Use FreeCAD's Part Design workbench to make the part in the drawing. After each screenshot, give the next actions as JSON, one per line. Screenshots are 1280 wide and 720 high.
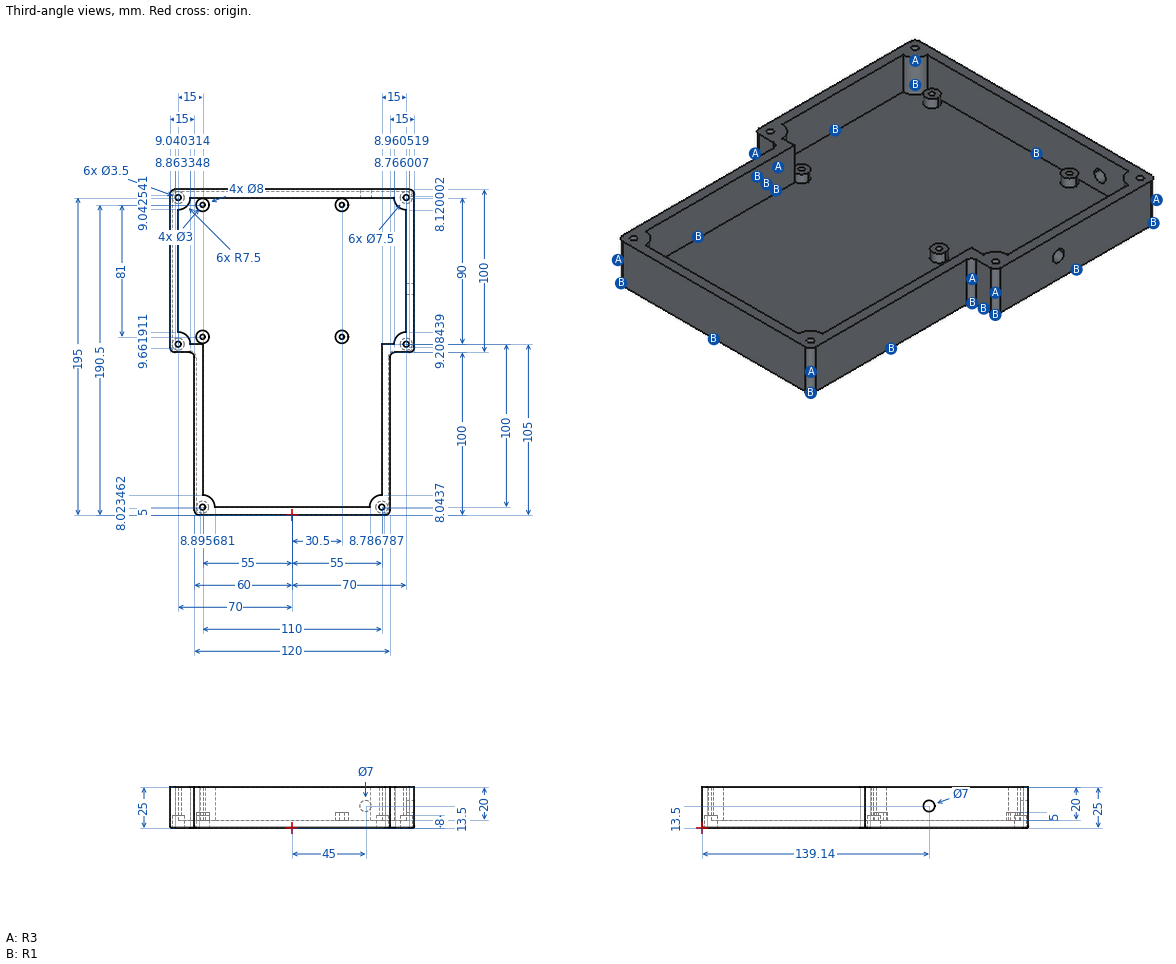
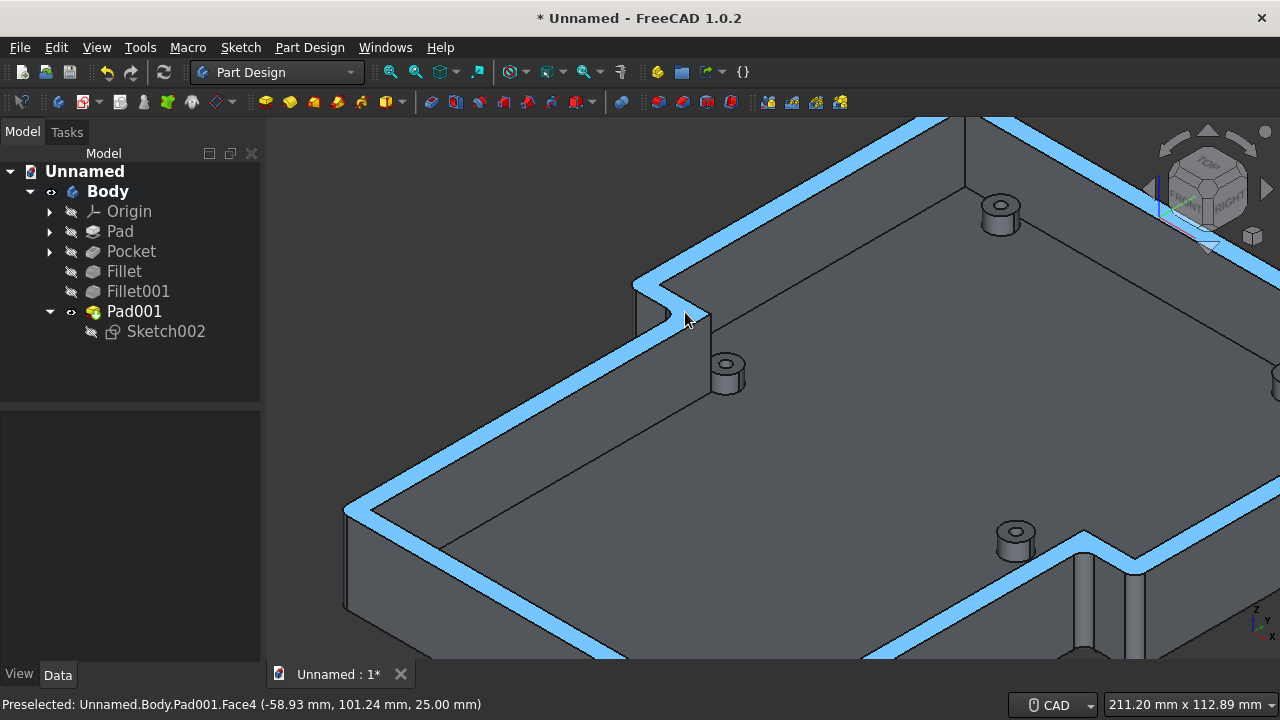
{"action": "left_click", "coordinate": [684, 313]}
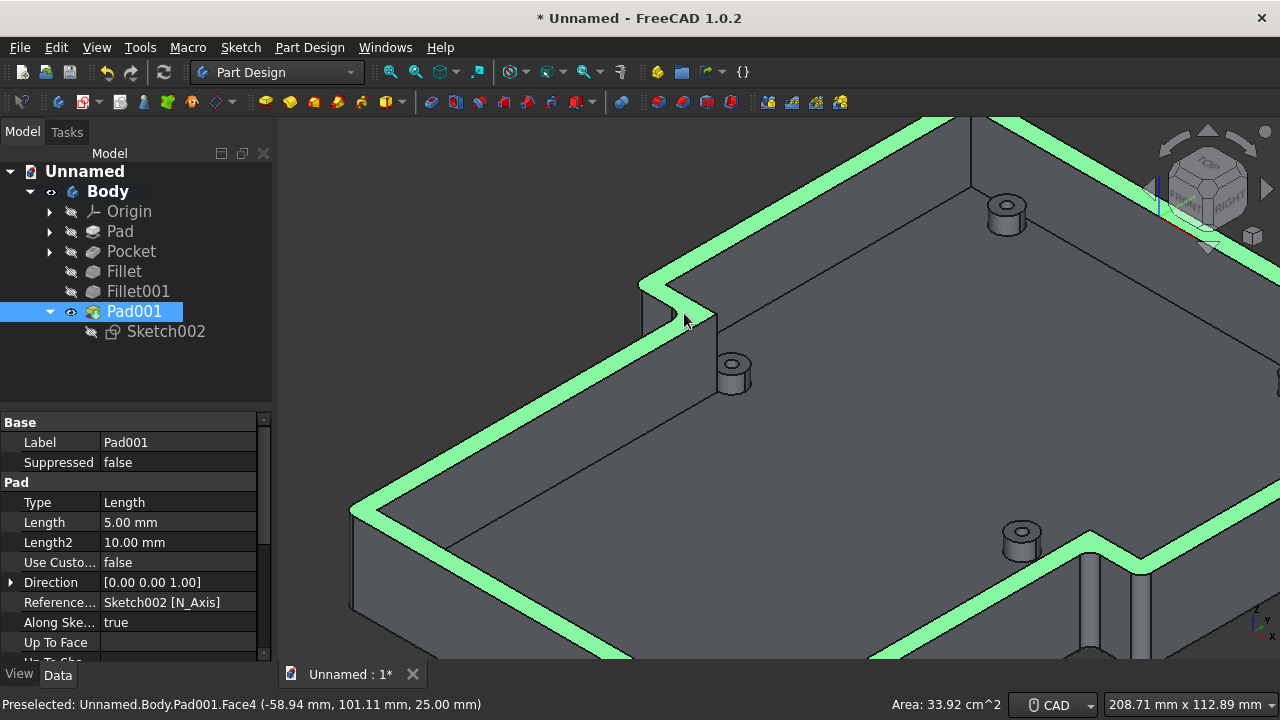
{"action": "left_click", "coordinate": [84, 102]}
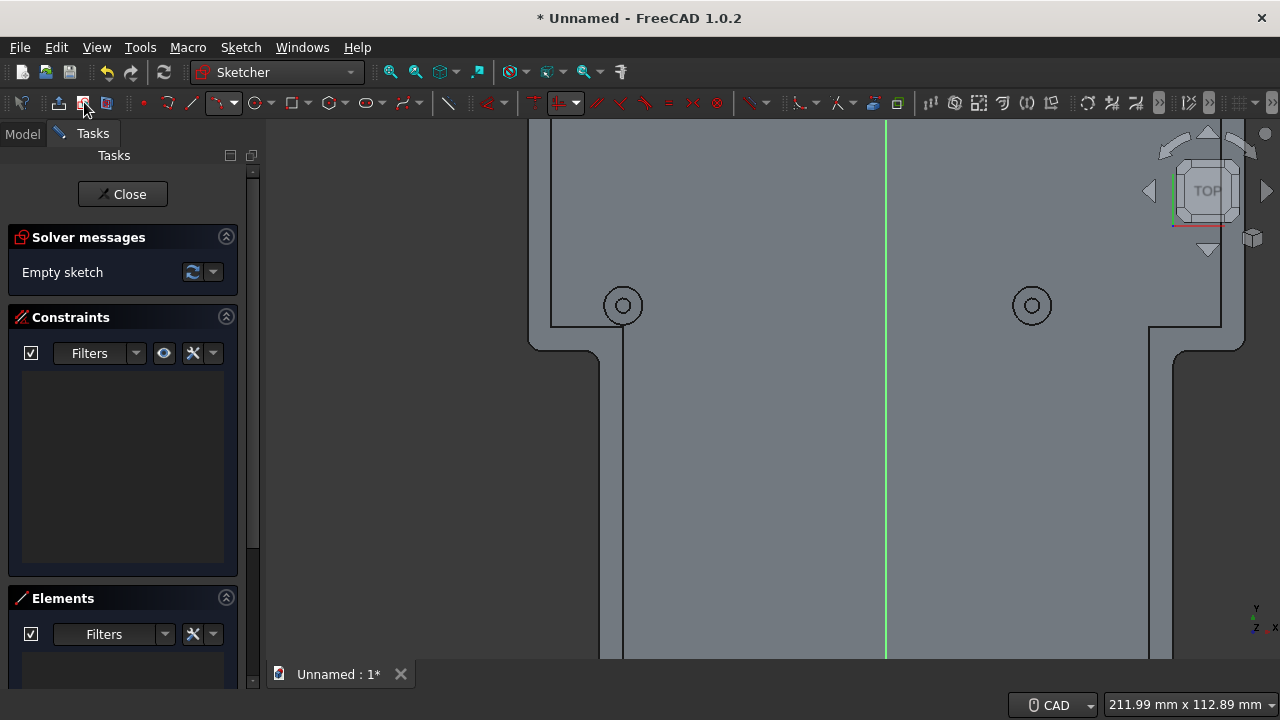
{"action": "scroll", "coordinate": [599, 407], "scroll_direction": "down", "scroll_amount": 5}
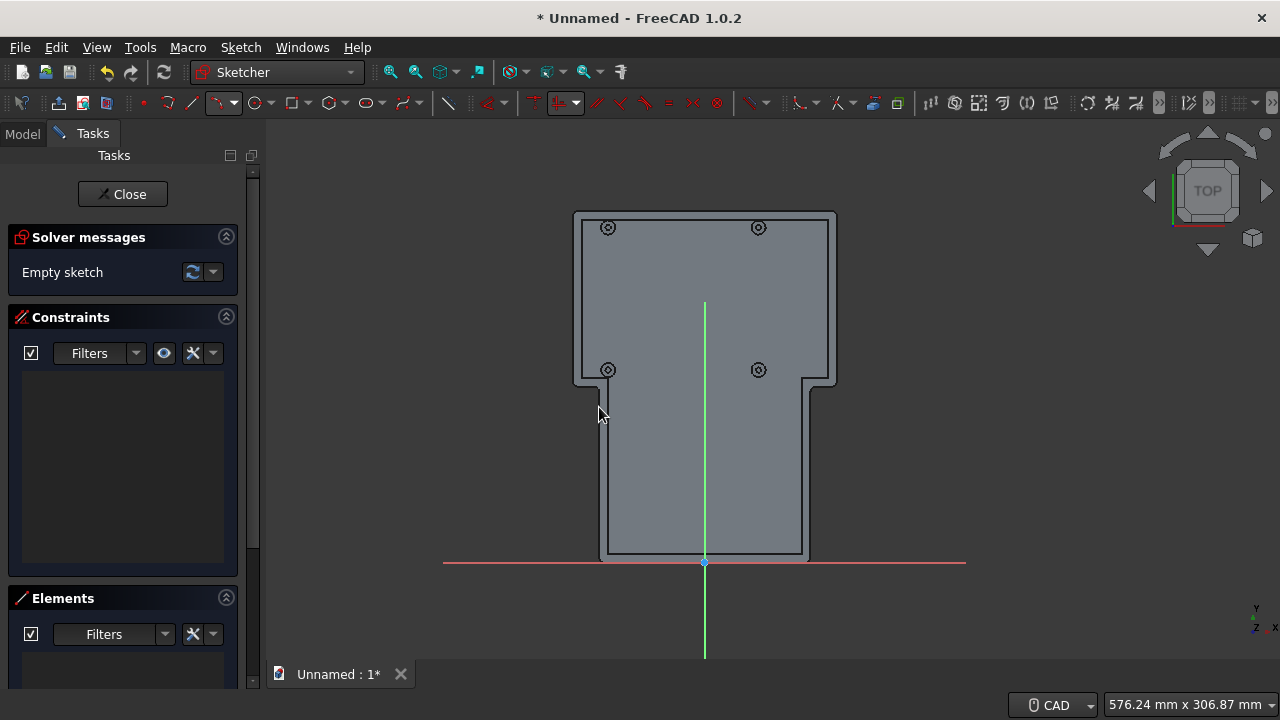
{"action": "key", "text": "g m"}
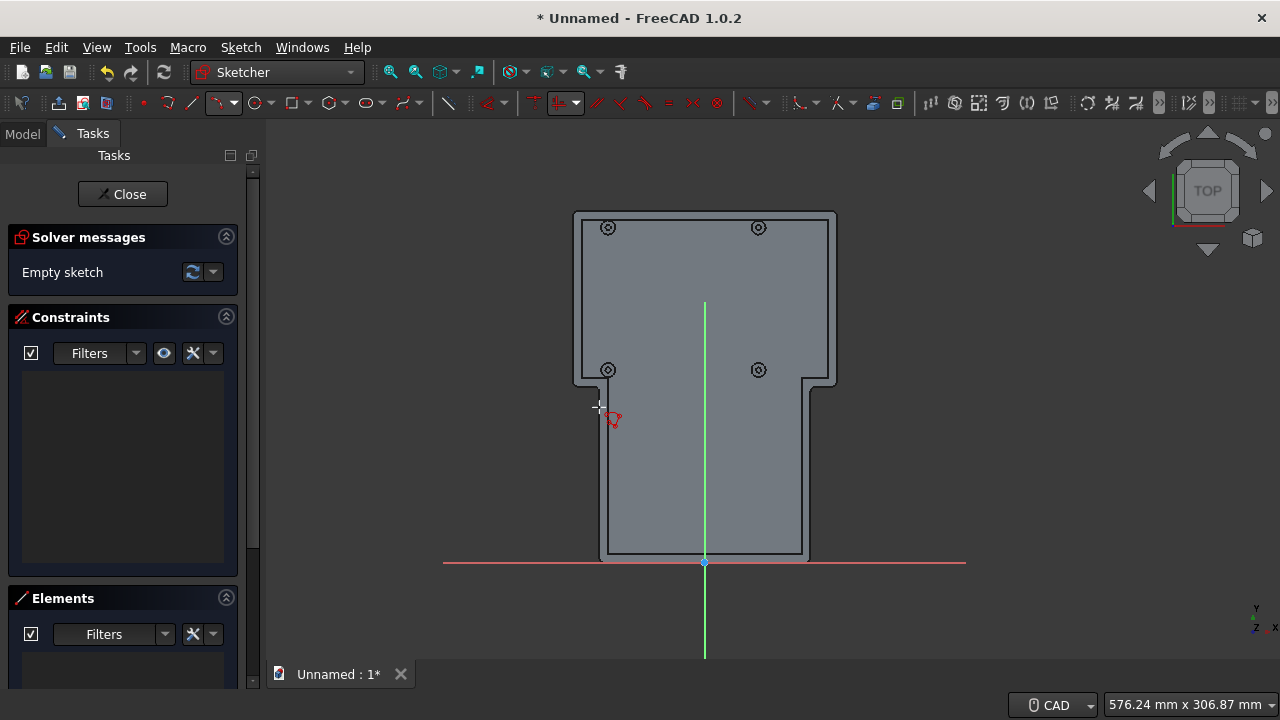
{"action": "left_click", "coordinate": [595, 217]}
{"action": "left_click", "coordinate": [579, 217]}
{"action": "left_click", "coordinate": [579, 232]}
{"action": "right_click", "coordinate": [579, 232]}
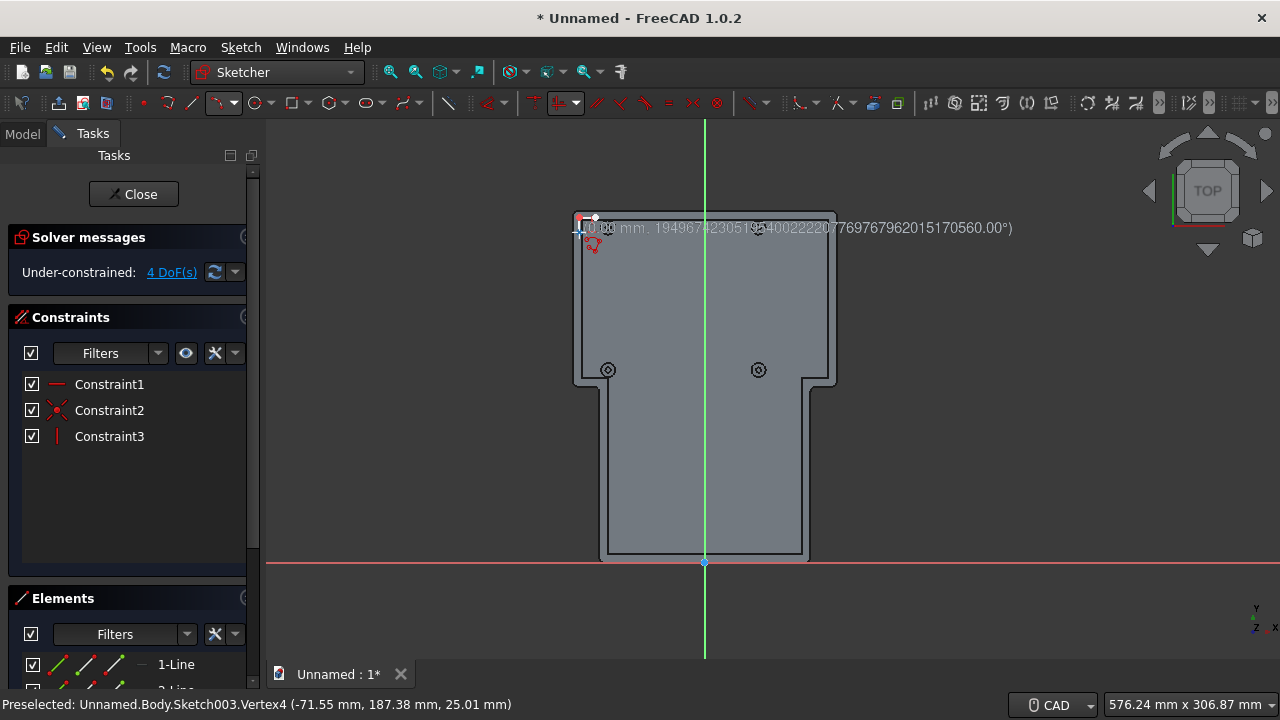
{"action": "key", "text": "g 3 a"}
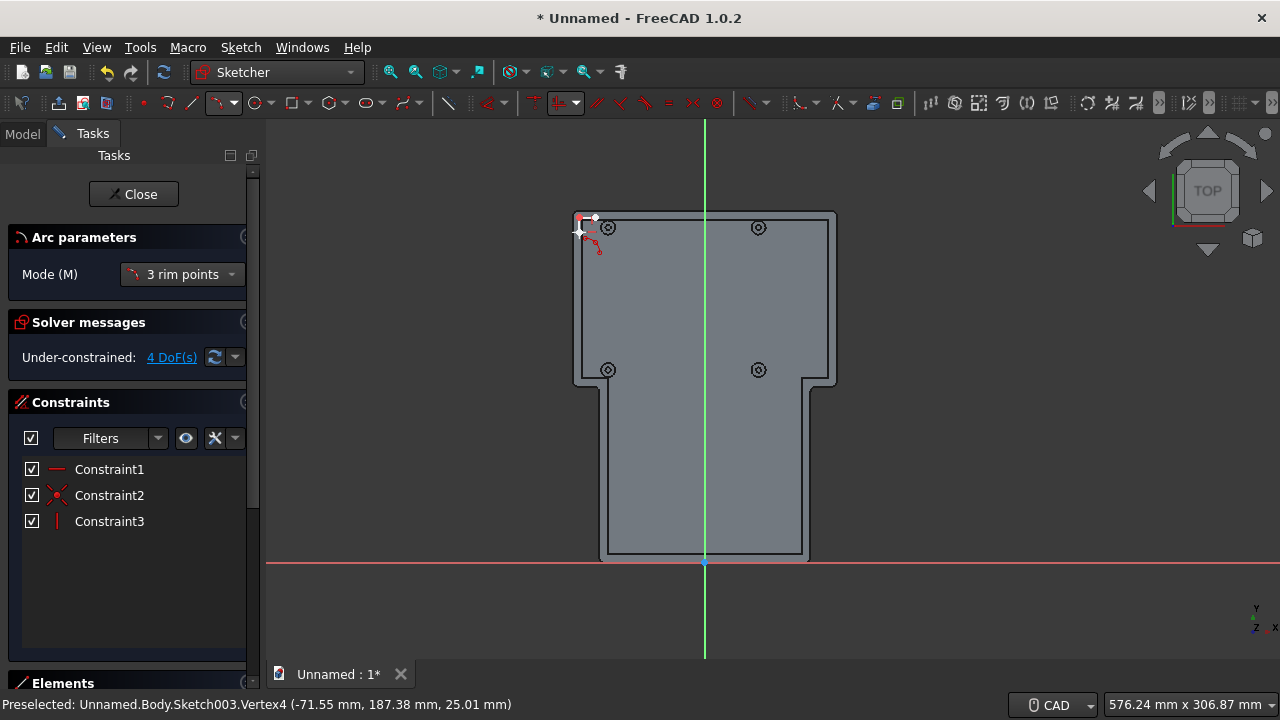
{"action": "scroll", "coordinate": [579, 232], "scroll_direction": "up", "scroll_amount": 4}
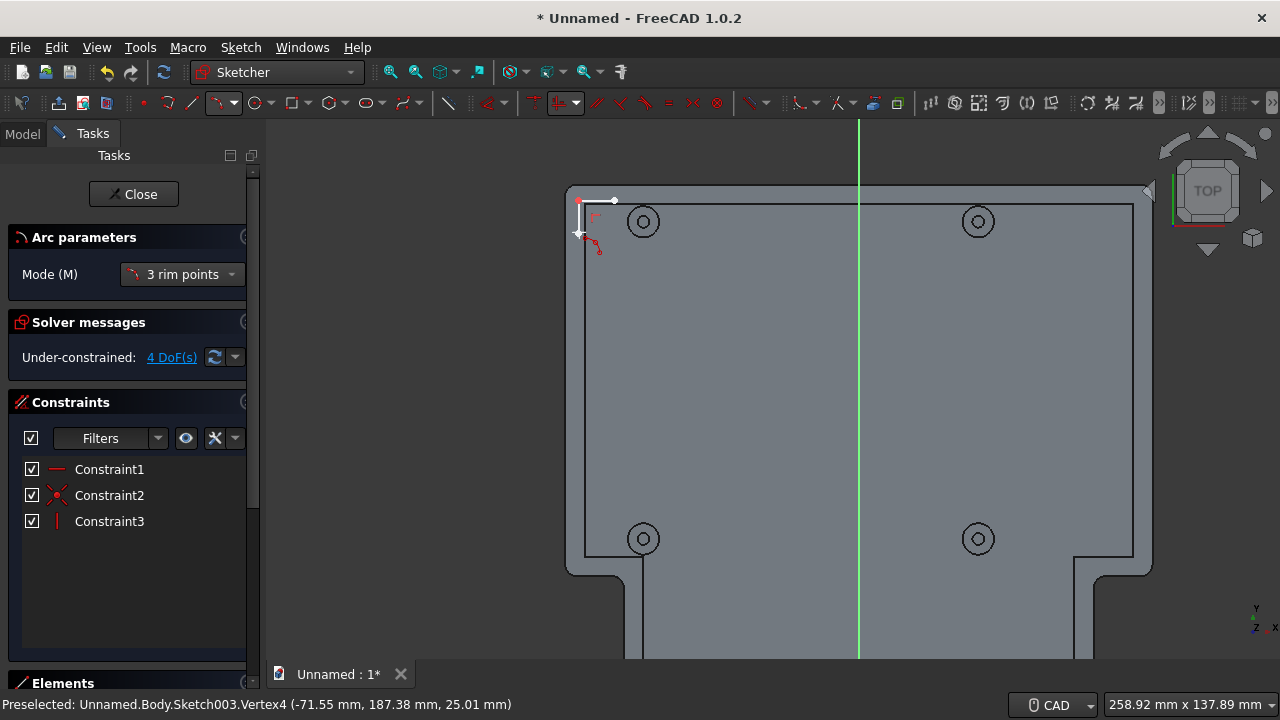
{"action": "left_click", "coordinate": [579, 234]}
{"action": "left_click", "coordinate": [614, 201]}
{"action": "left_click", "coordinate": [605, 225]}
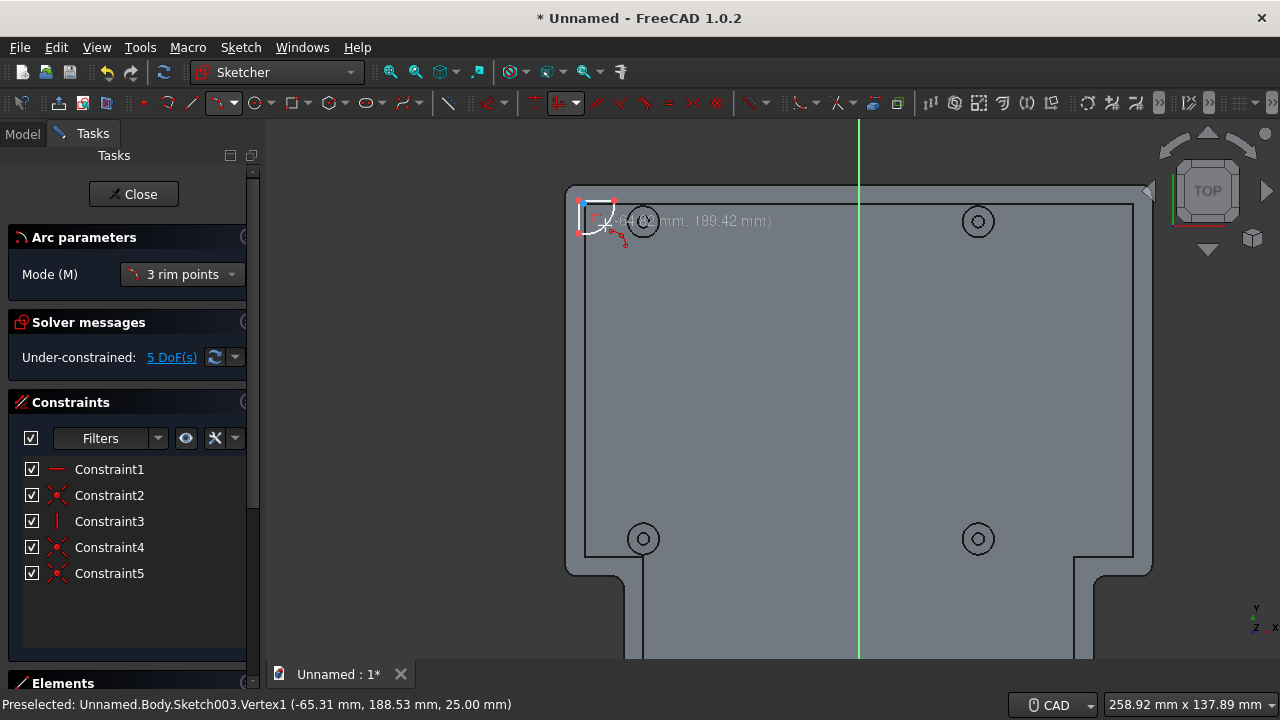
{"action": "key", "text": "g m"}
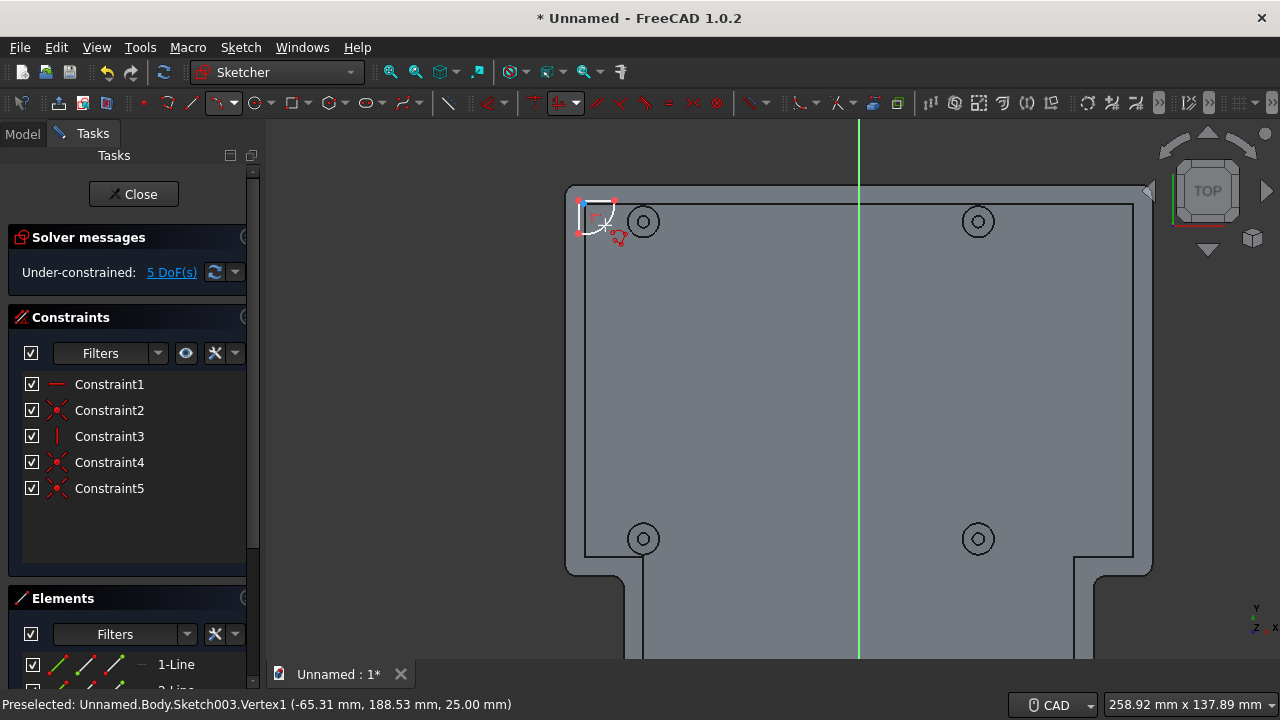
{"action": "scroll", "coordinate": [579, 231], "scroll_direction": "down", "scroll_amount": 4}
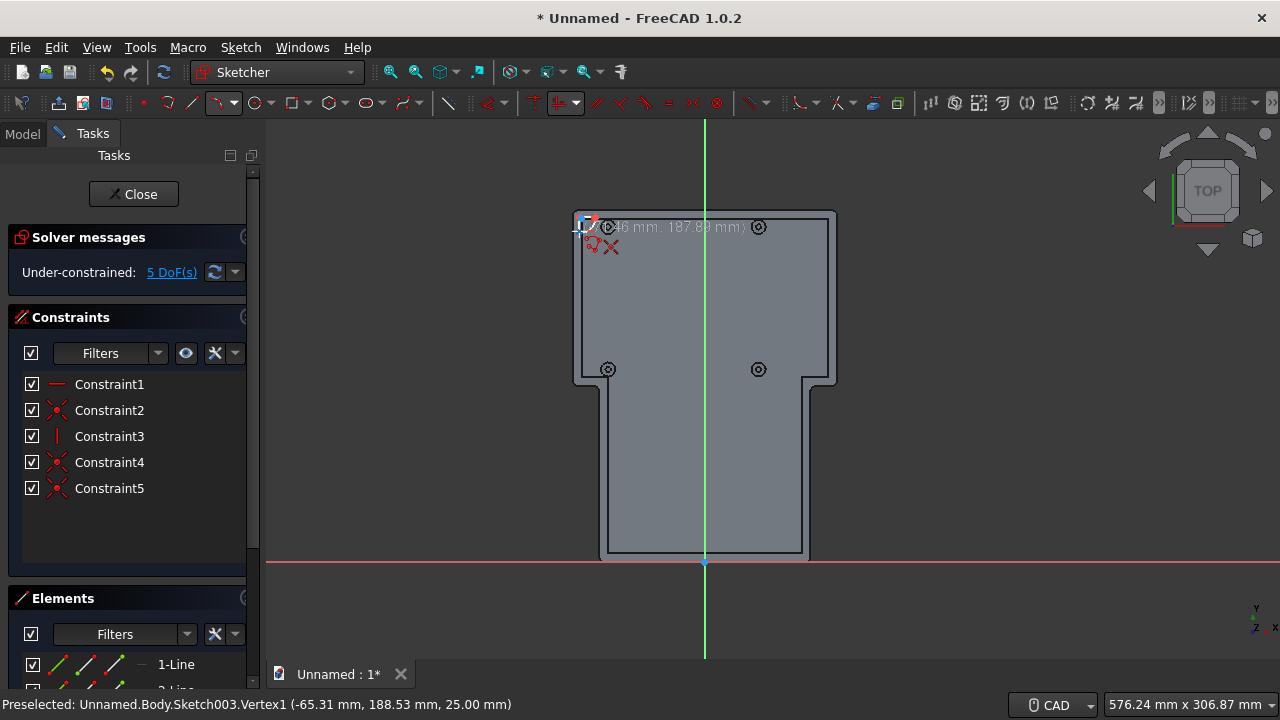
{"action": "left_click", "coordinate": [831, 232]}
{"action": "left_click", "coordinate": [831, 218]}
{"action": "left_click", "coordinate": [815, 218]}
{"action": "right_click", "coordinate": [815, 218]}